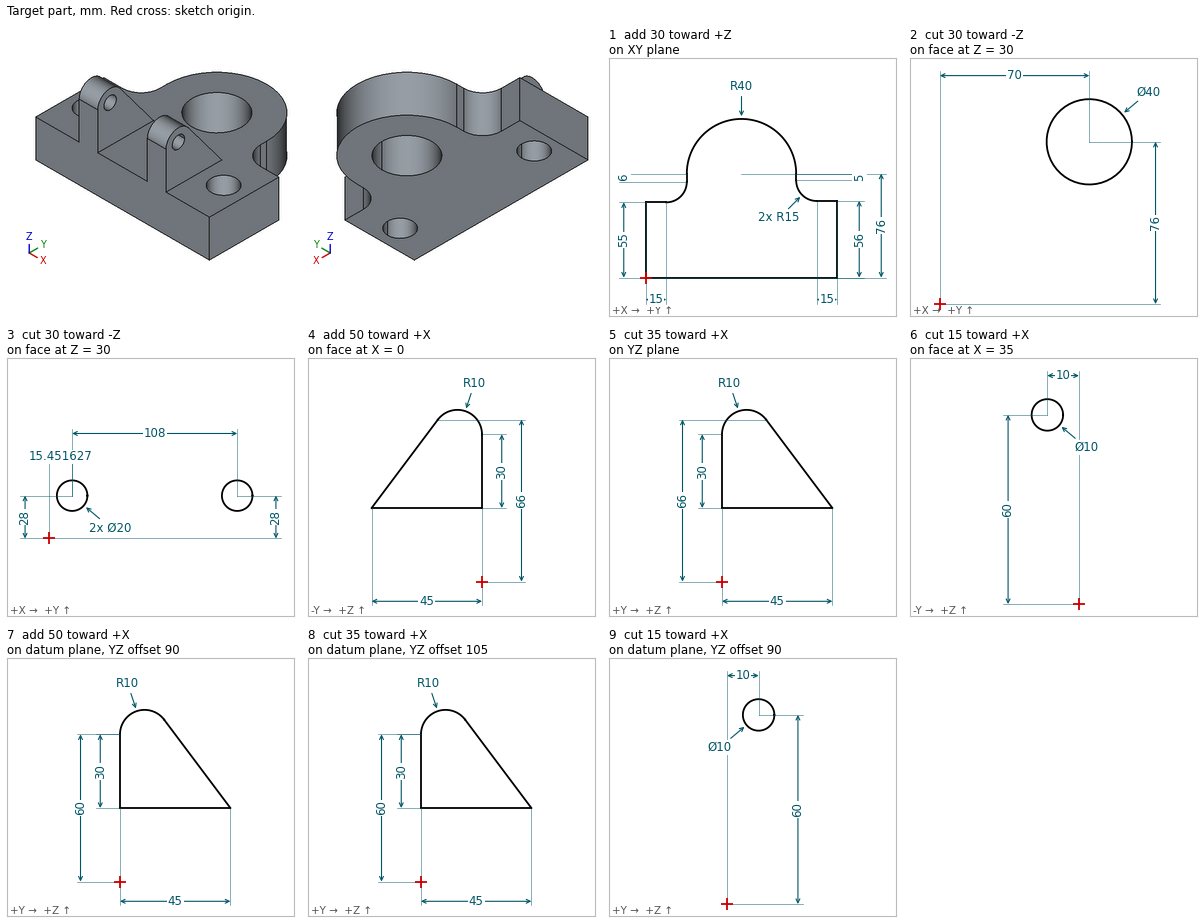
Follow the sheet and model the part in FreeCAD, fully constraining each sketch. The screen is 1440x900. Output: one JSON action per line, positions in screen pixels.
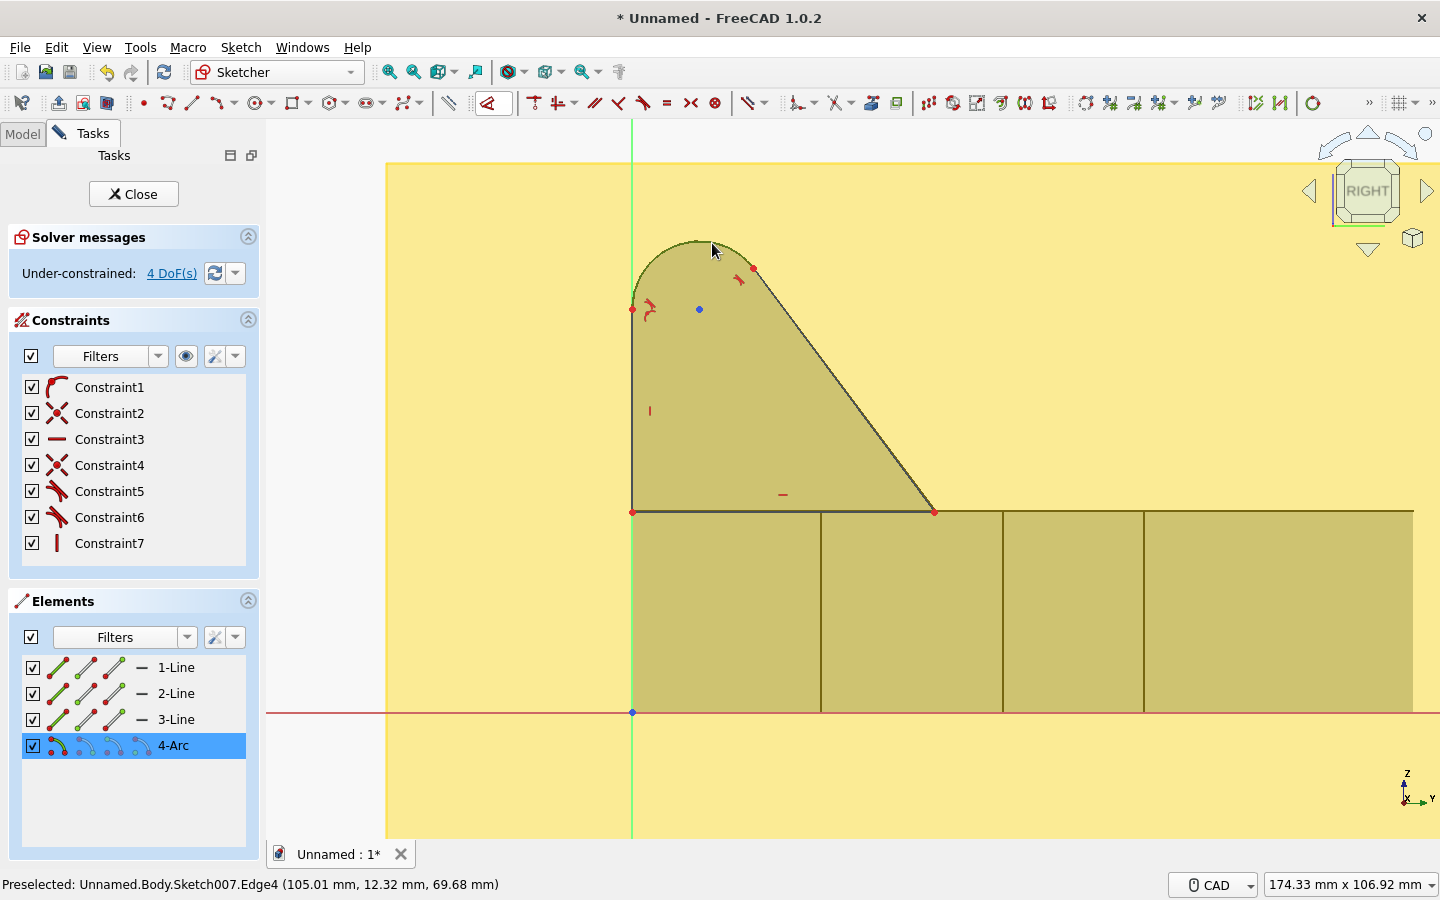
{"action": "key", "text": "k r"}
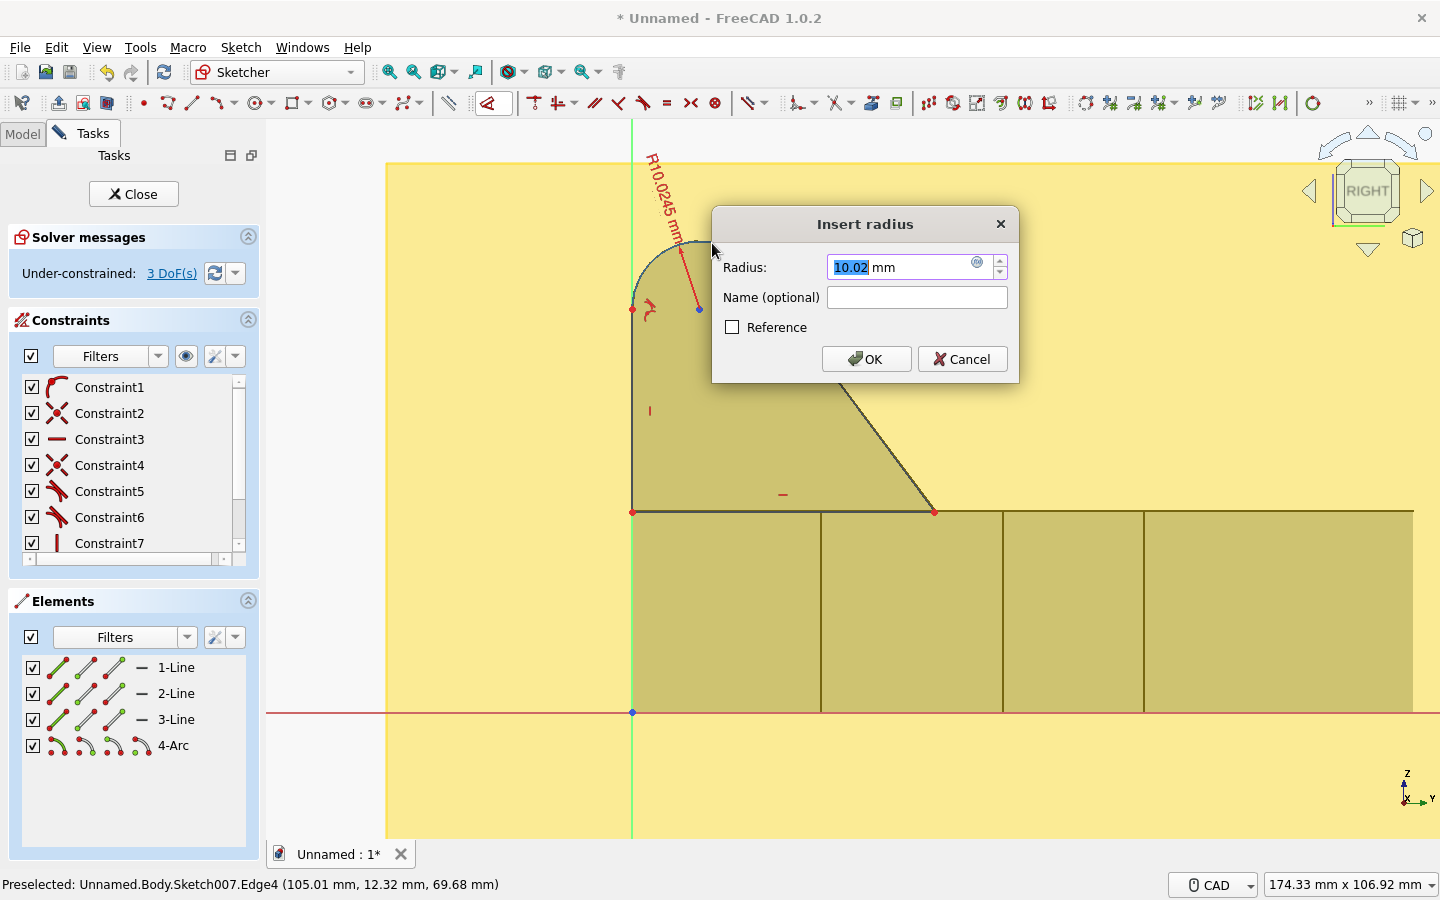
{"action": "type", "text": "10"}
{"action": "key", "text": "Return"}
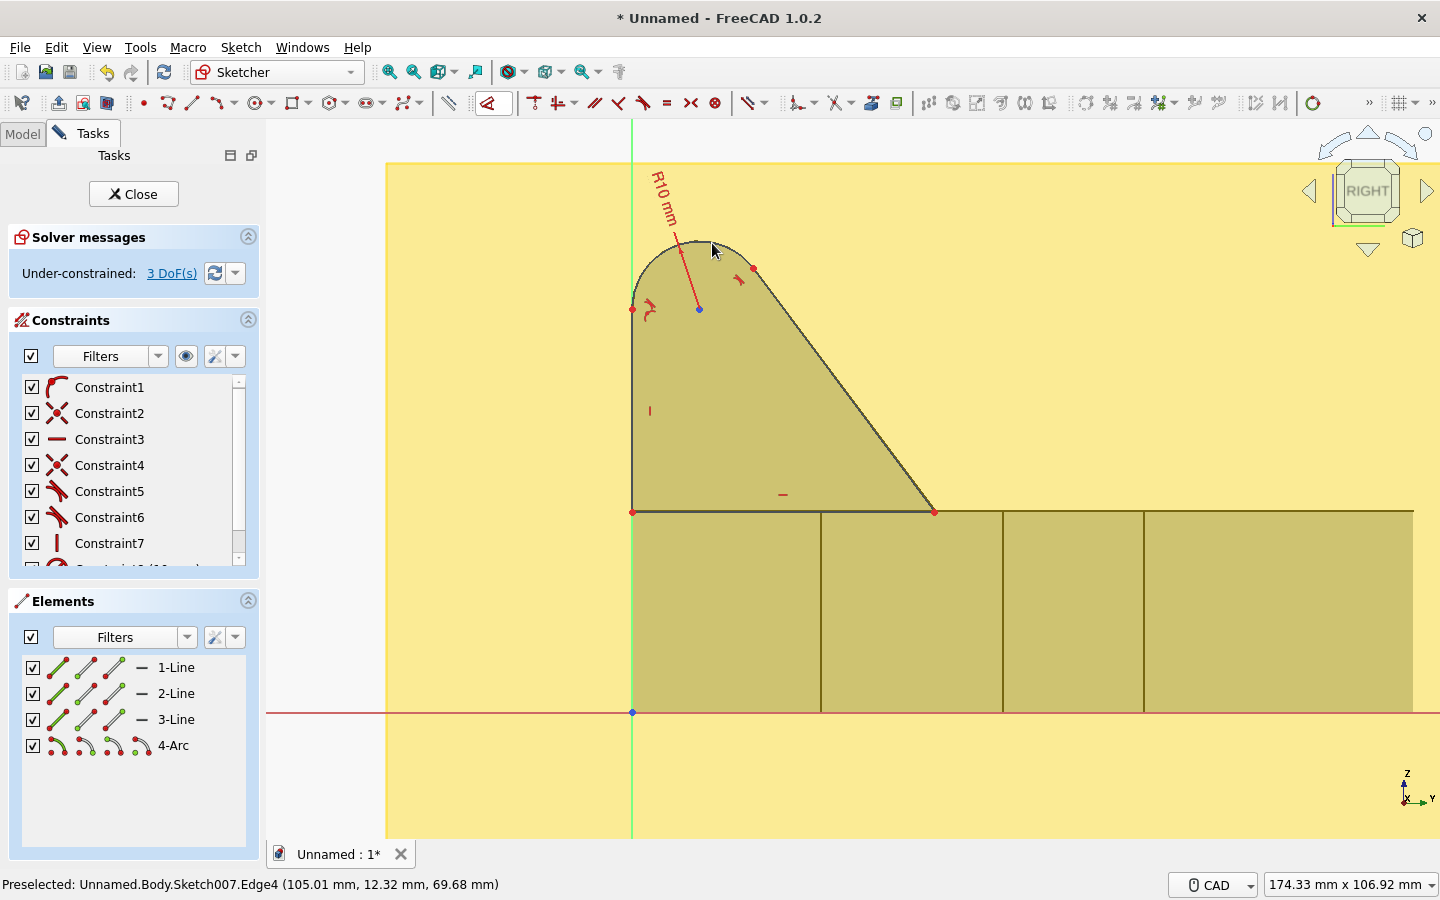
{"action": "left_click", "coordinate": [632, 370]}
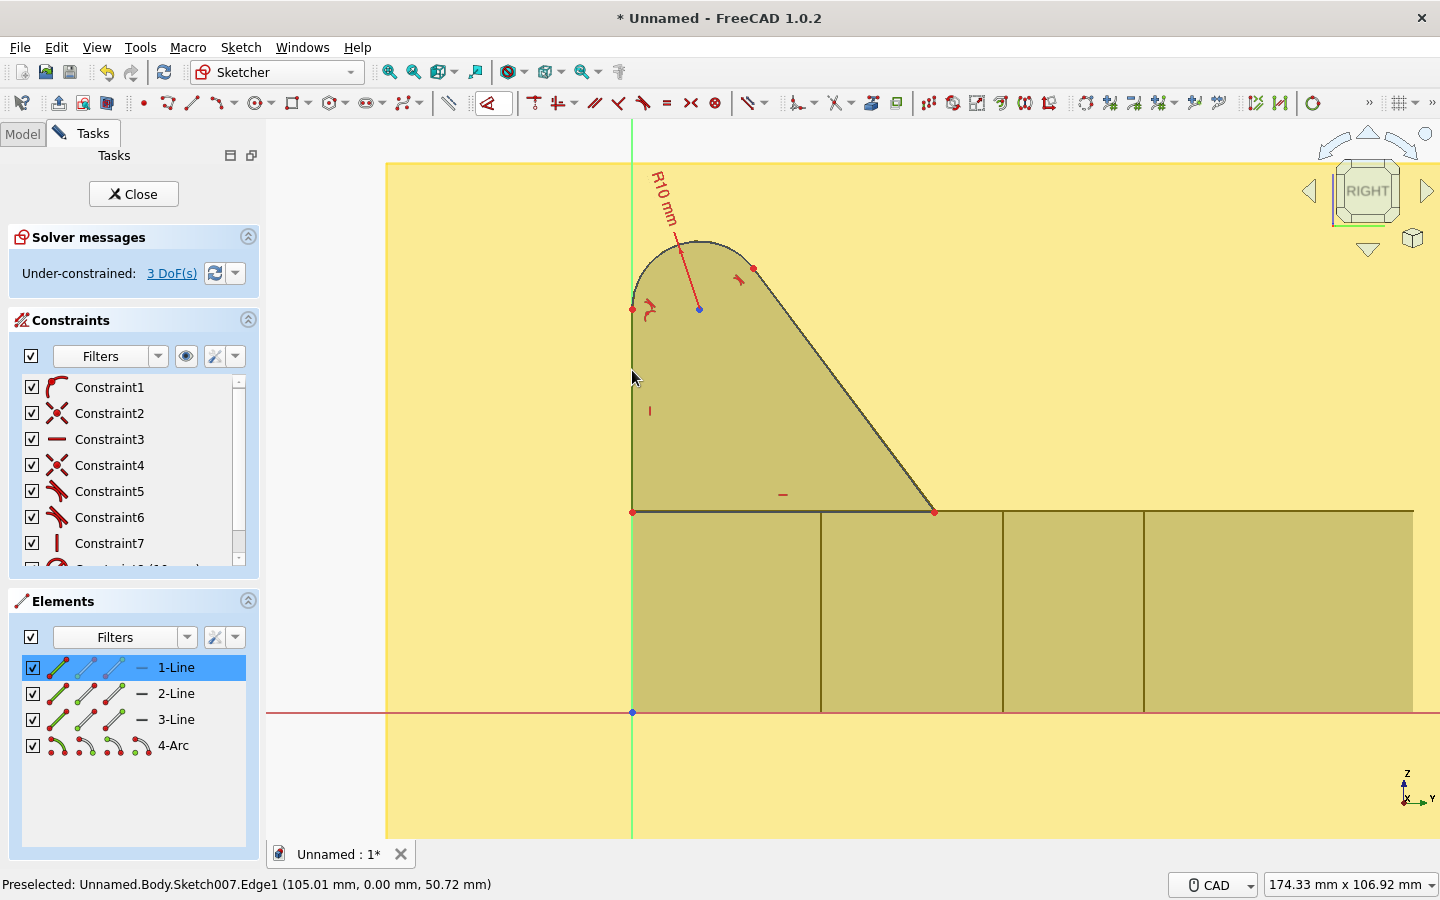
{"action": "key", "text": "i"}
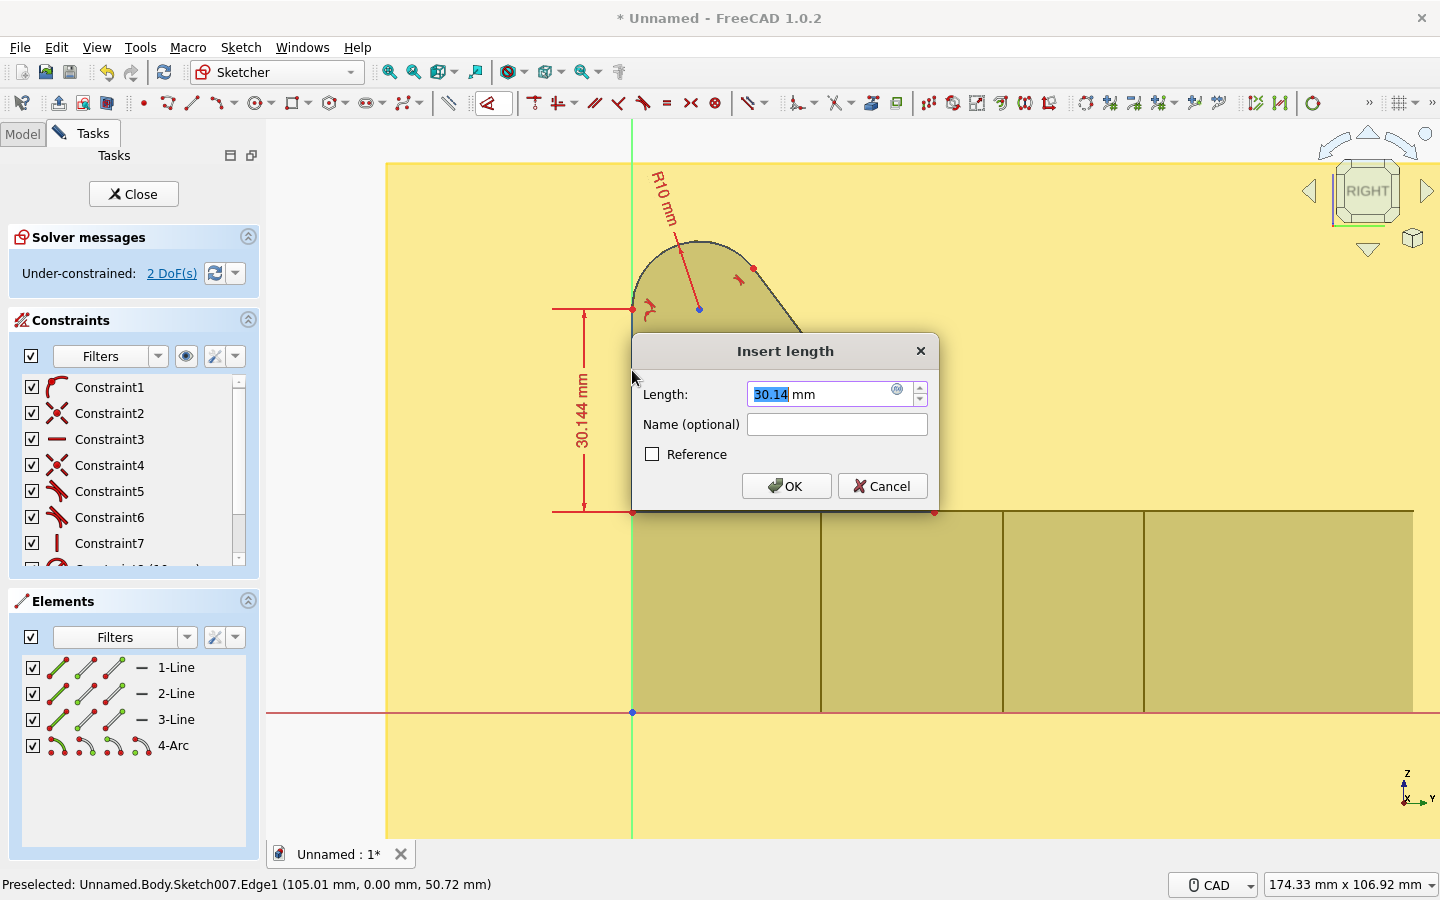
{"action": "type", "text": "30"}
{"action": "key", "text": "Return"}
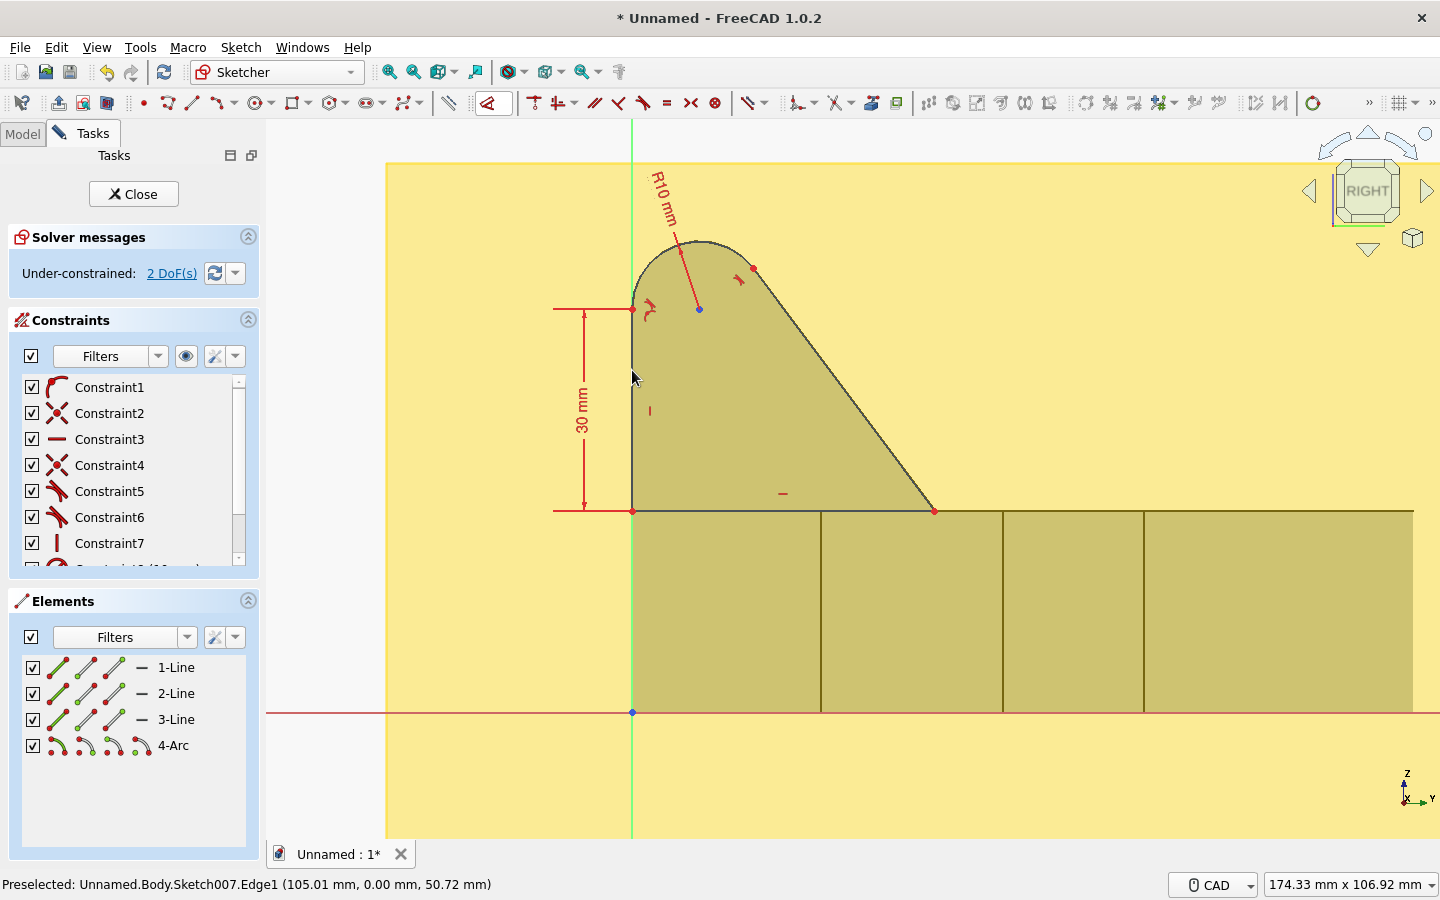
{"action": "left_click", "coordinate": [723, 511]}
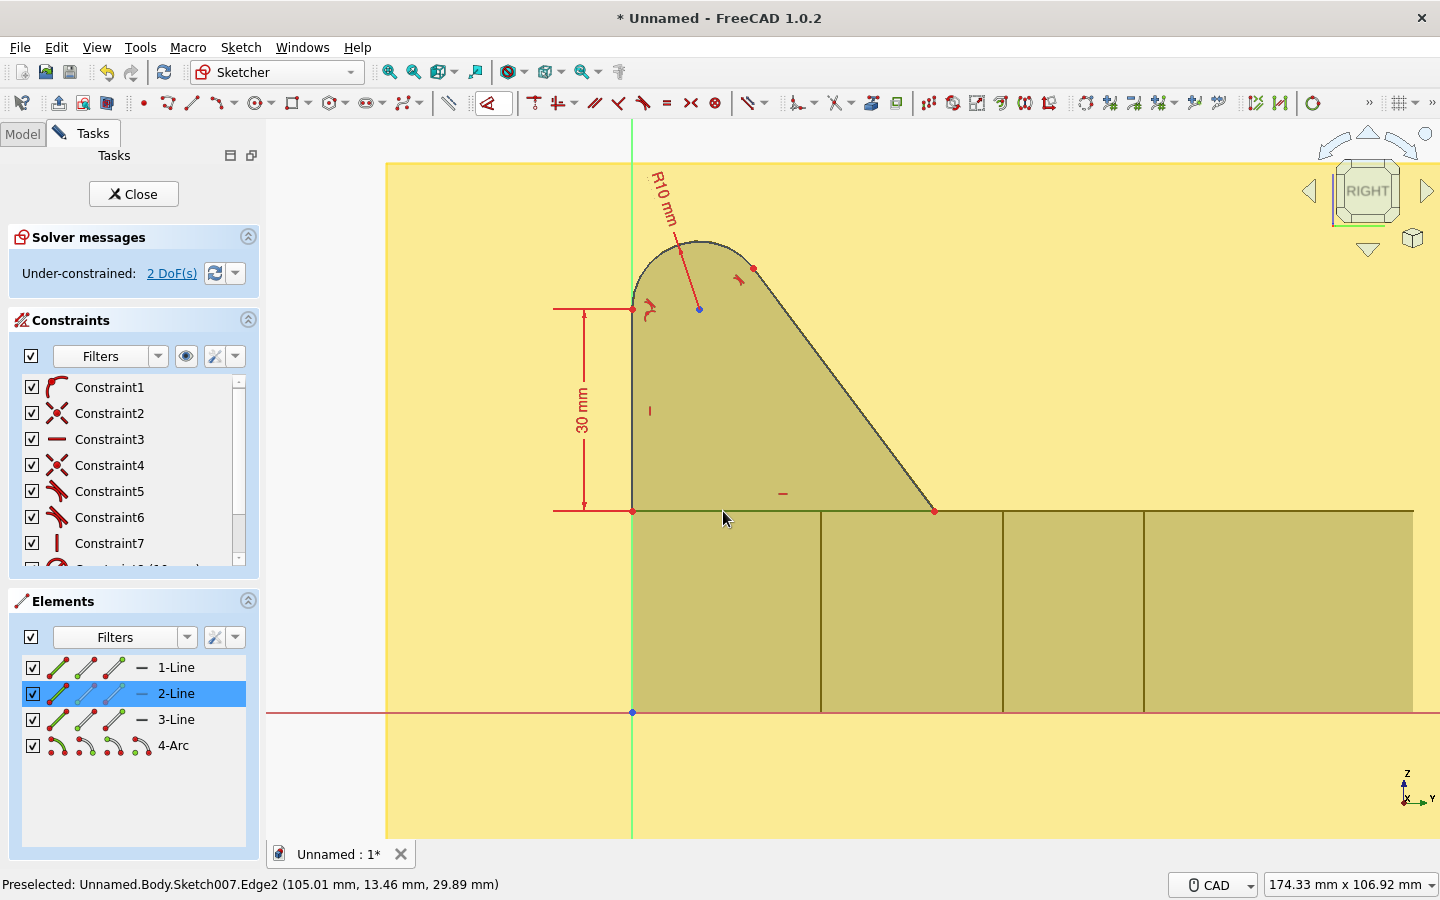
{"action": "key", "text": "l"}